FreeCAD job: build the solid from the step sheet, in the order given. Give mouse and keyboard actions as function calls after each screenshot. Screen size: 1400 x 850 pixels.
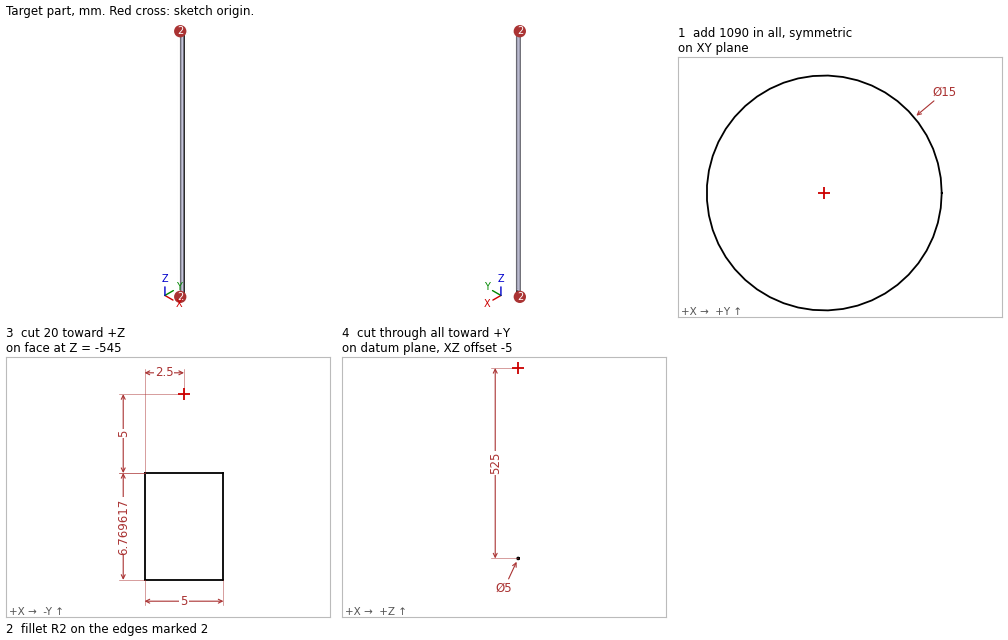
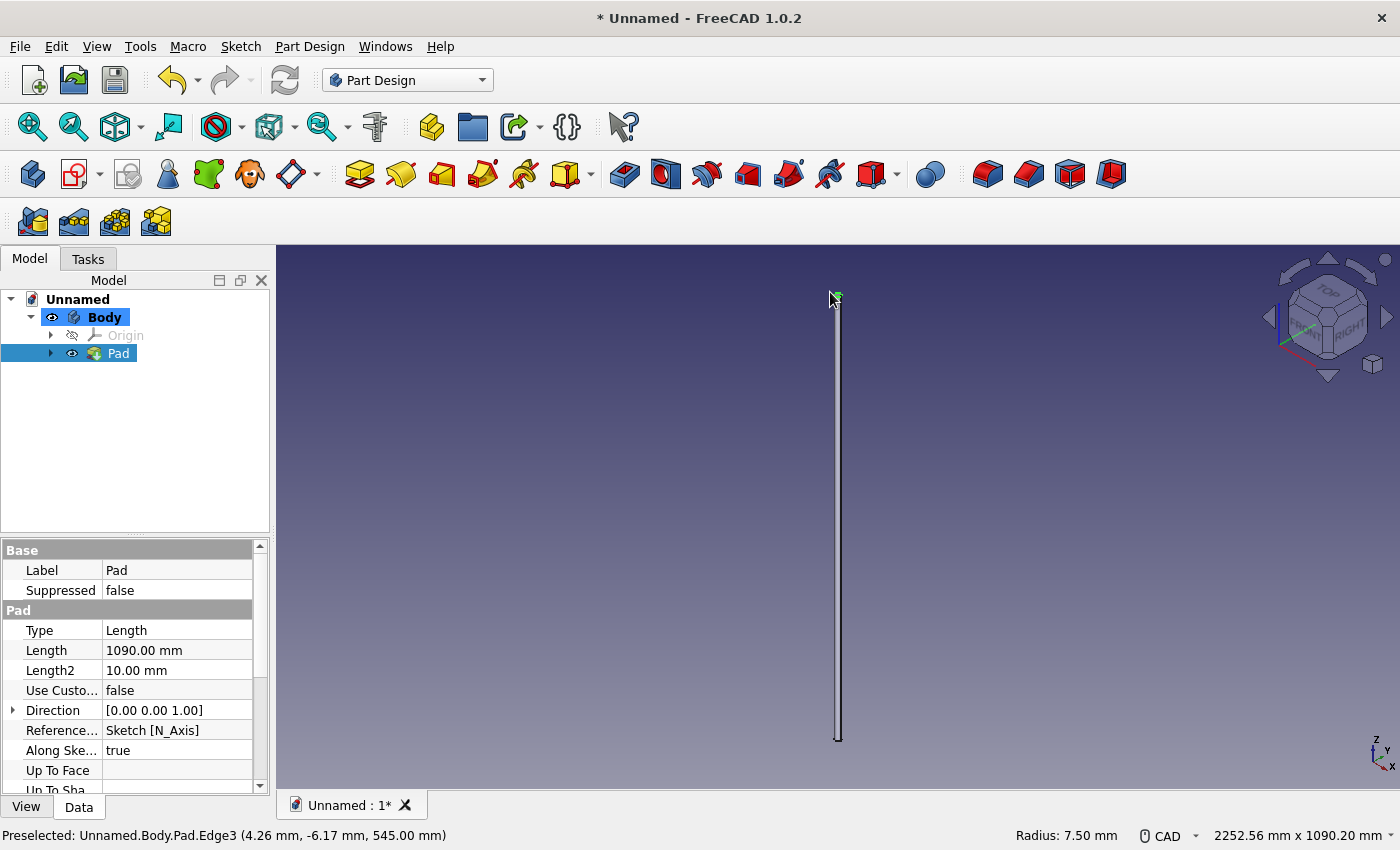
key(2)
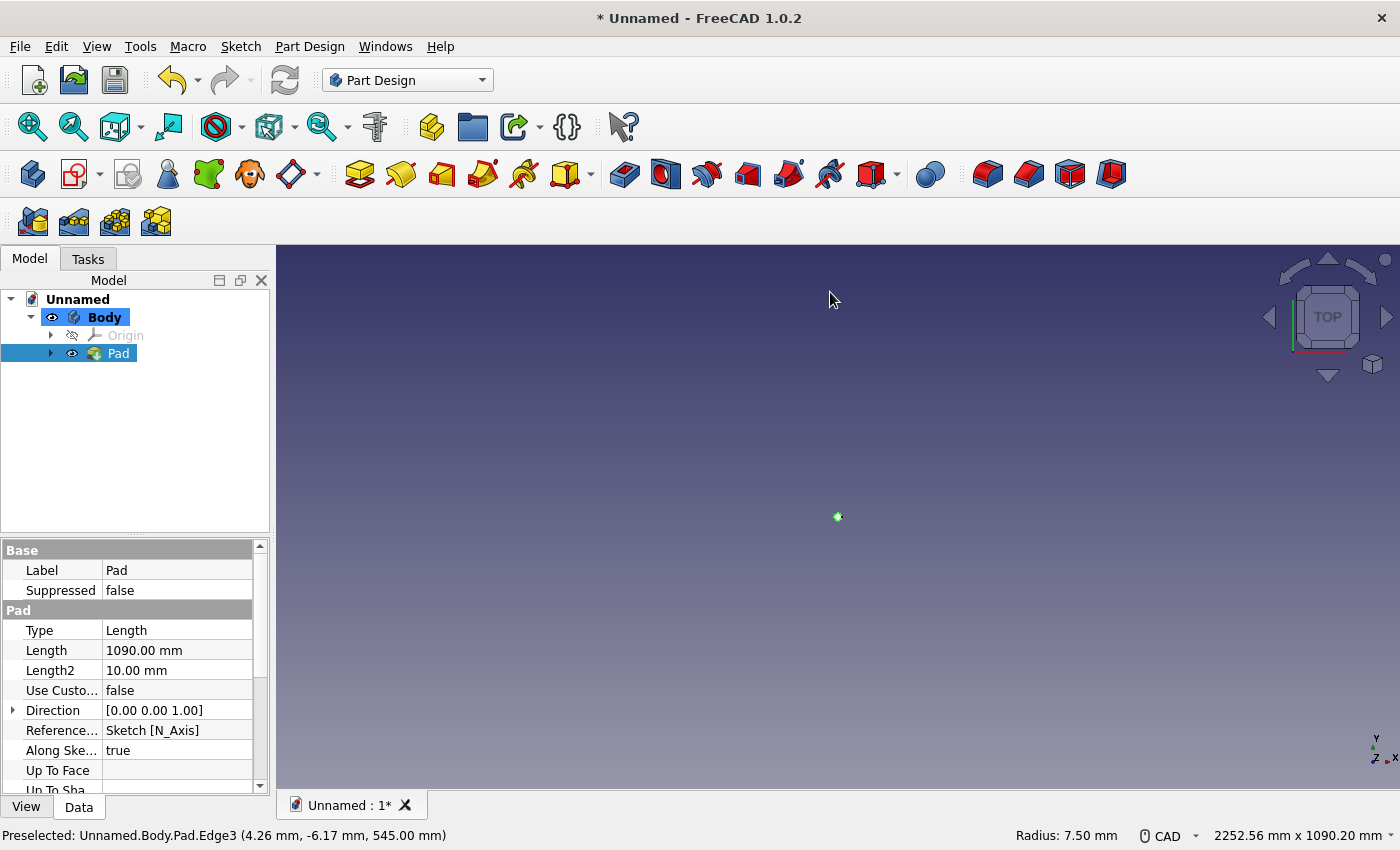
key(v)
key(f)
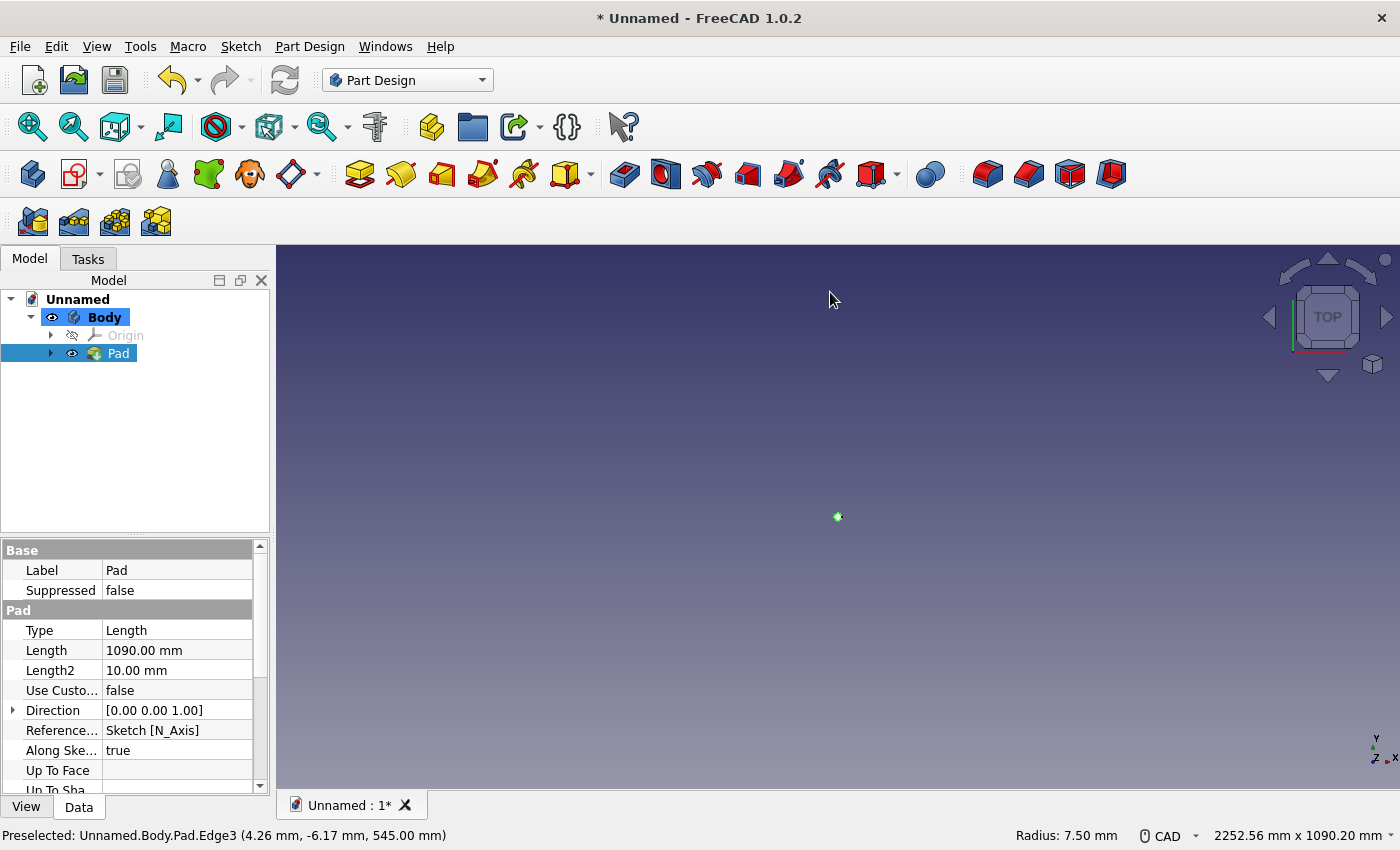
key(1)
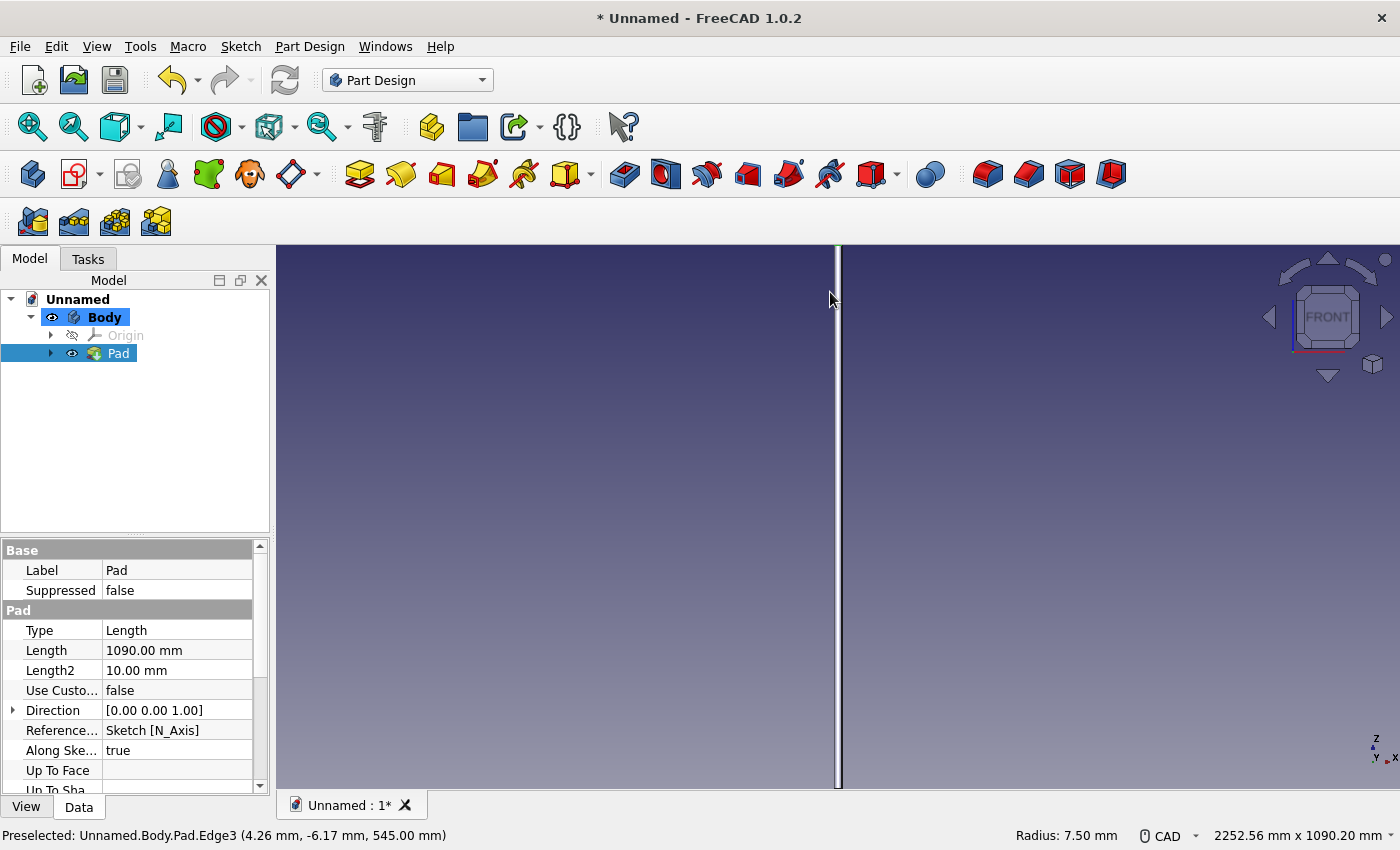
key(v)
key(f)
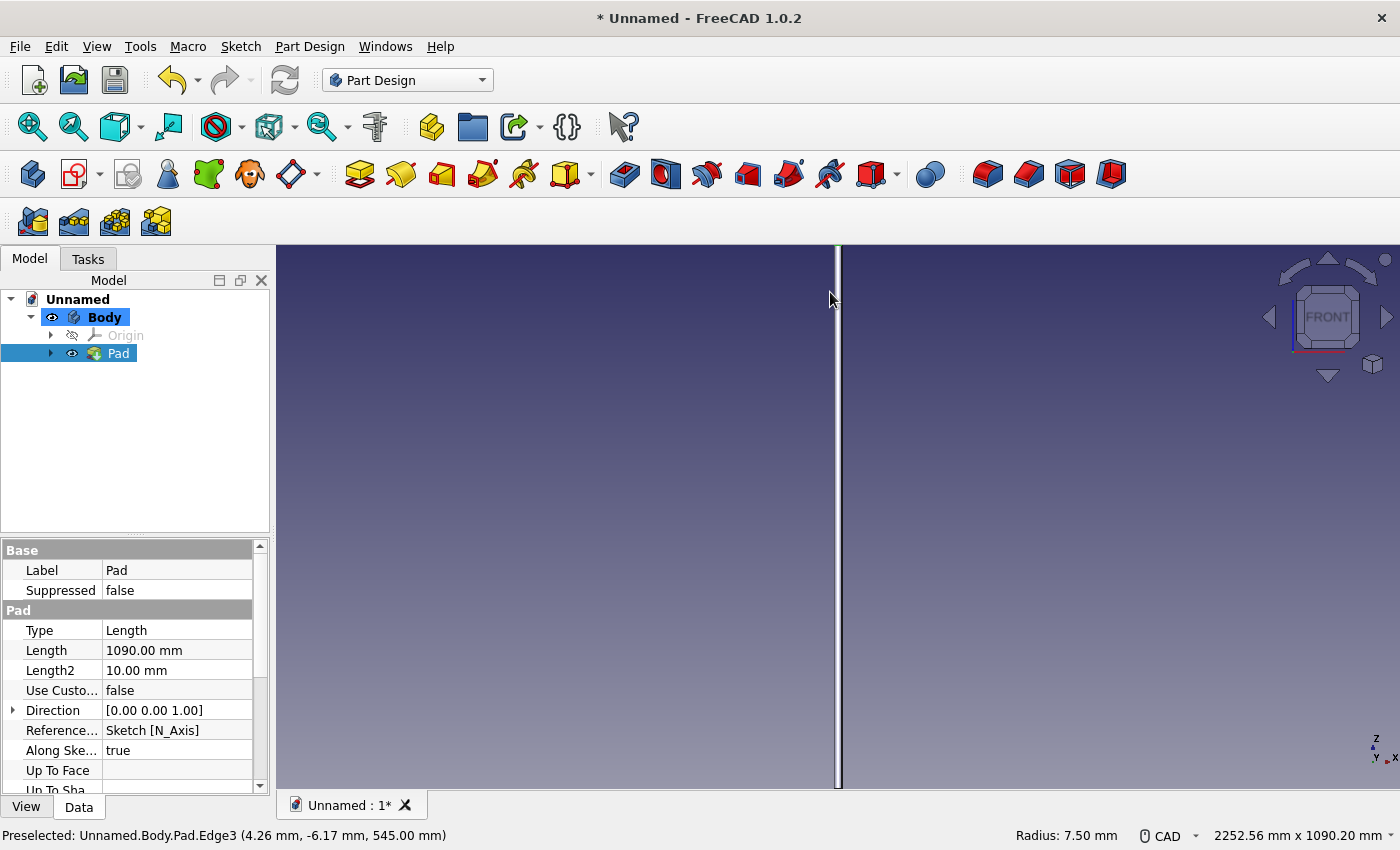
key(3)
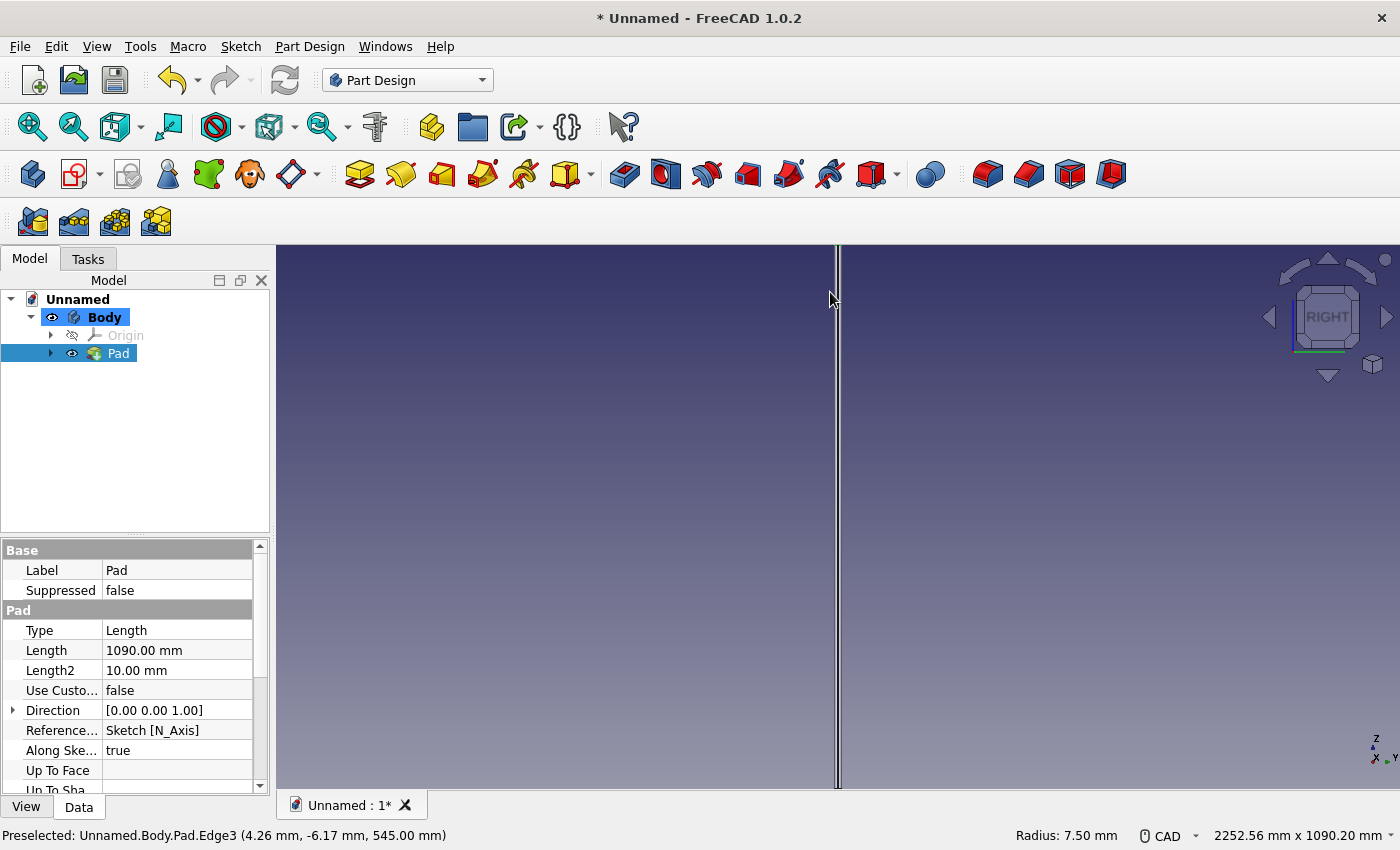
key(v)
key(f)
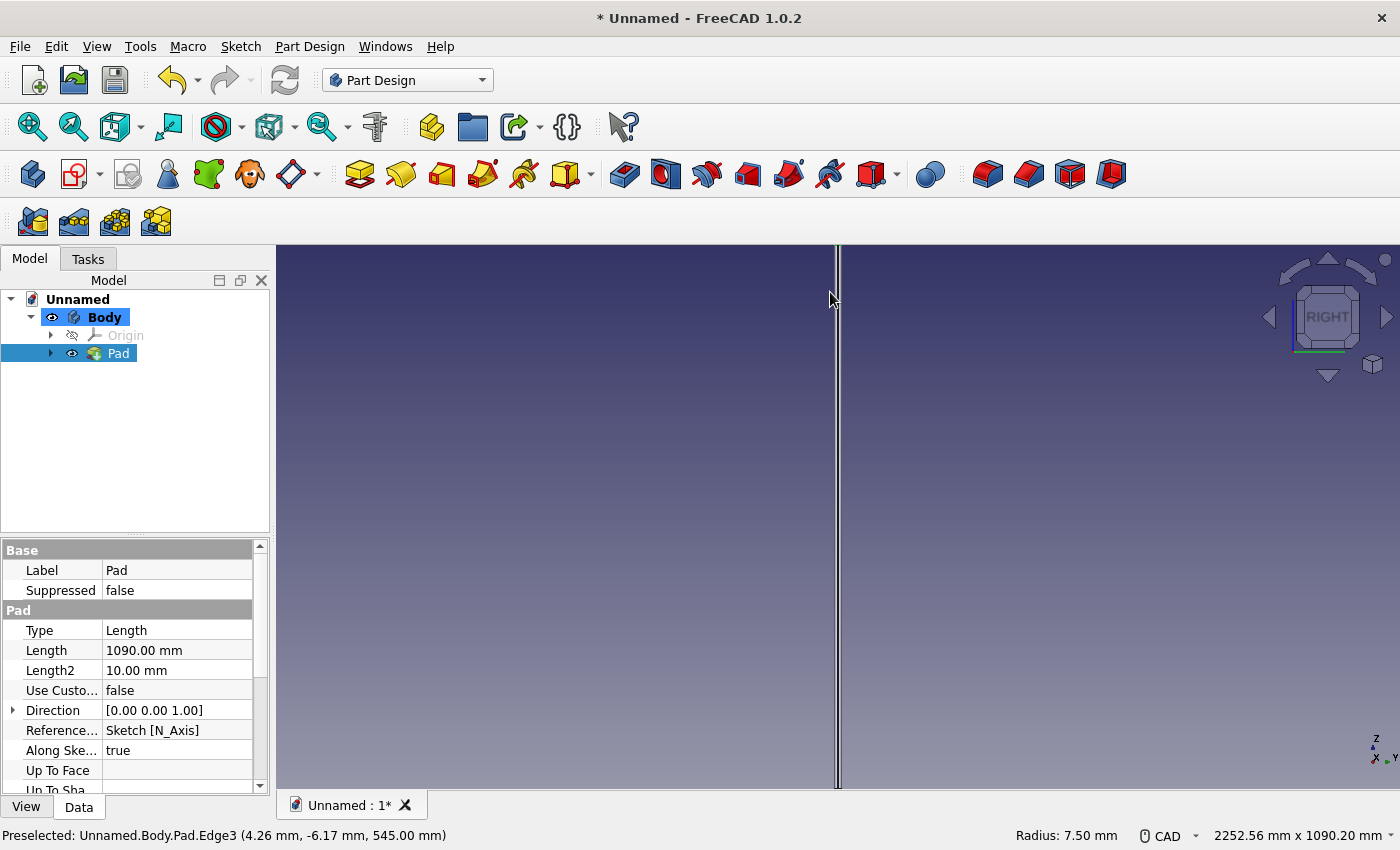
key(5)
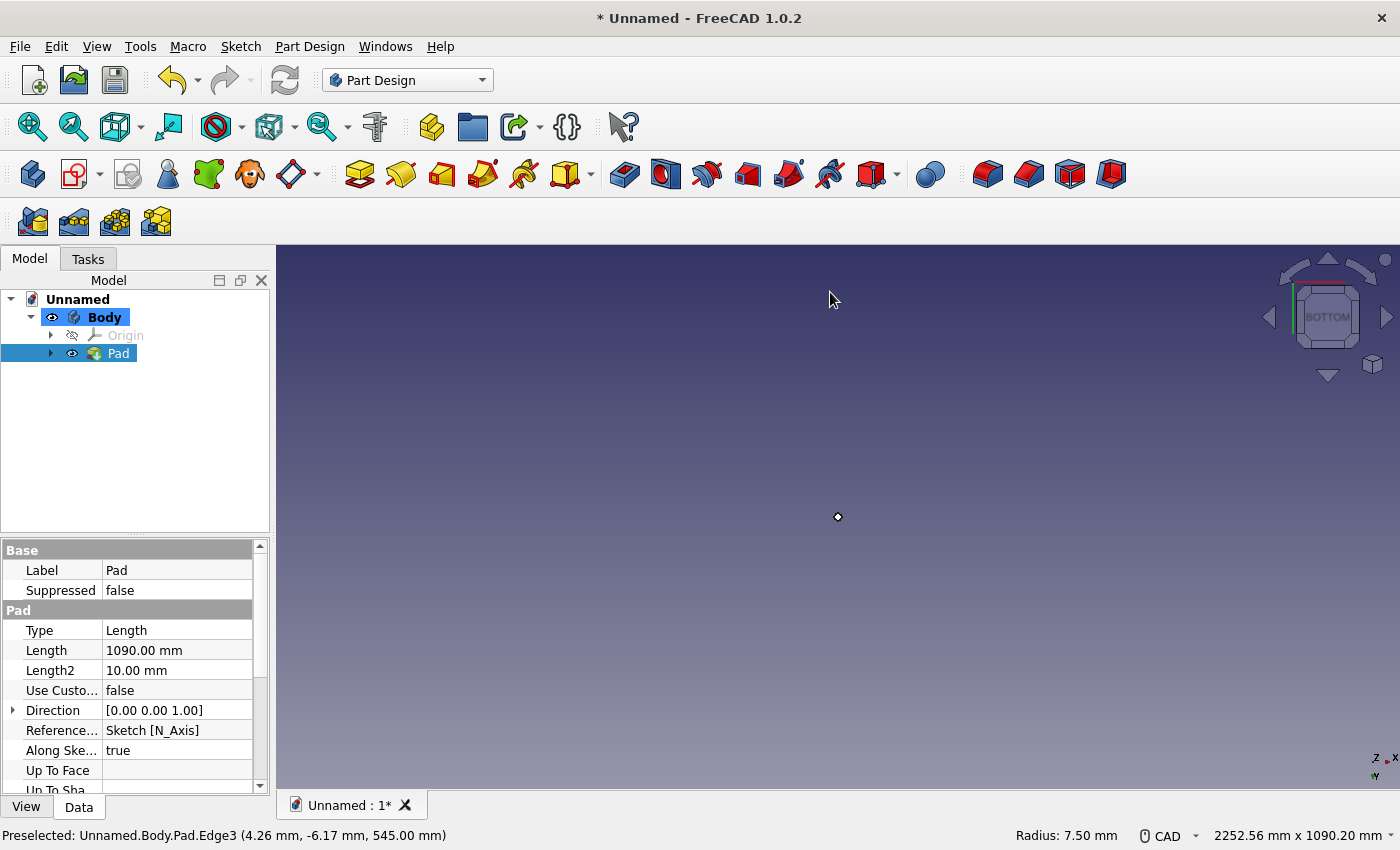
click(33, 128)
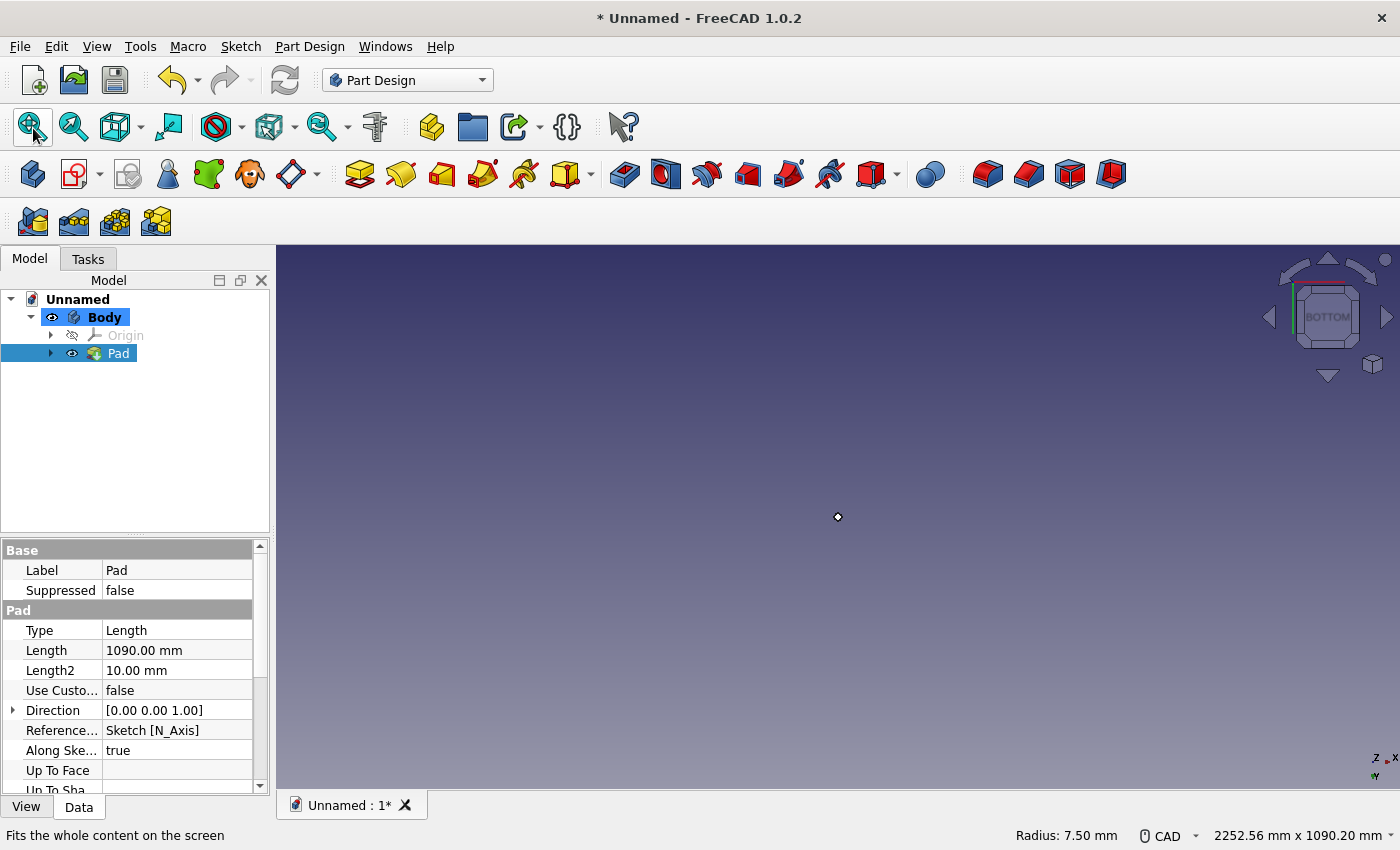
click(834, 516, ctrl)